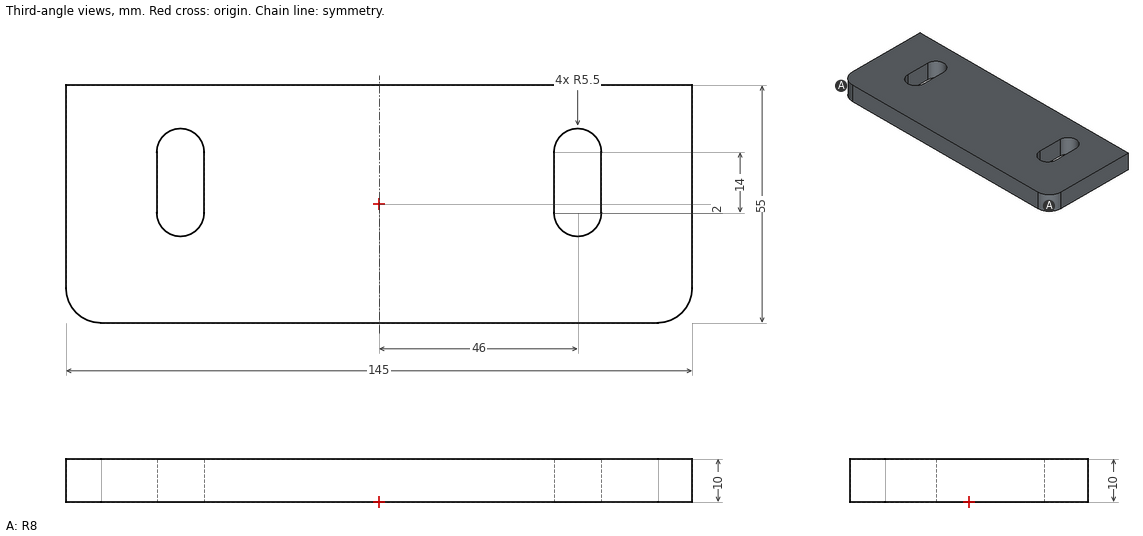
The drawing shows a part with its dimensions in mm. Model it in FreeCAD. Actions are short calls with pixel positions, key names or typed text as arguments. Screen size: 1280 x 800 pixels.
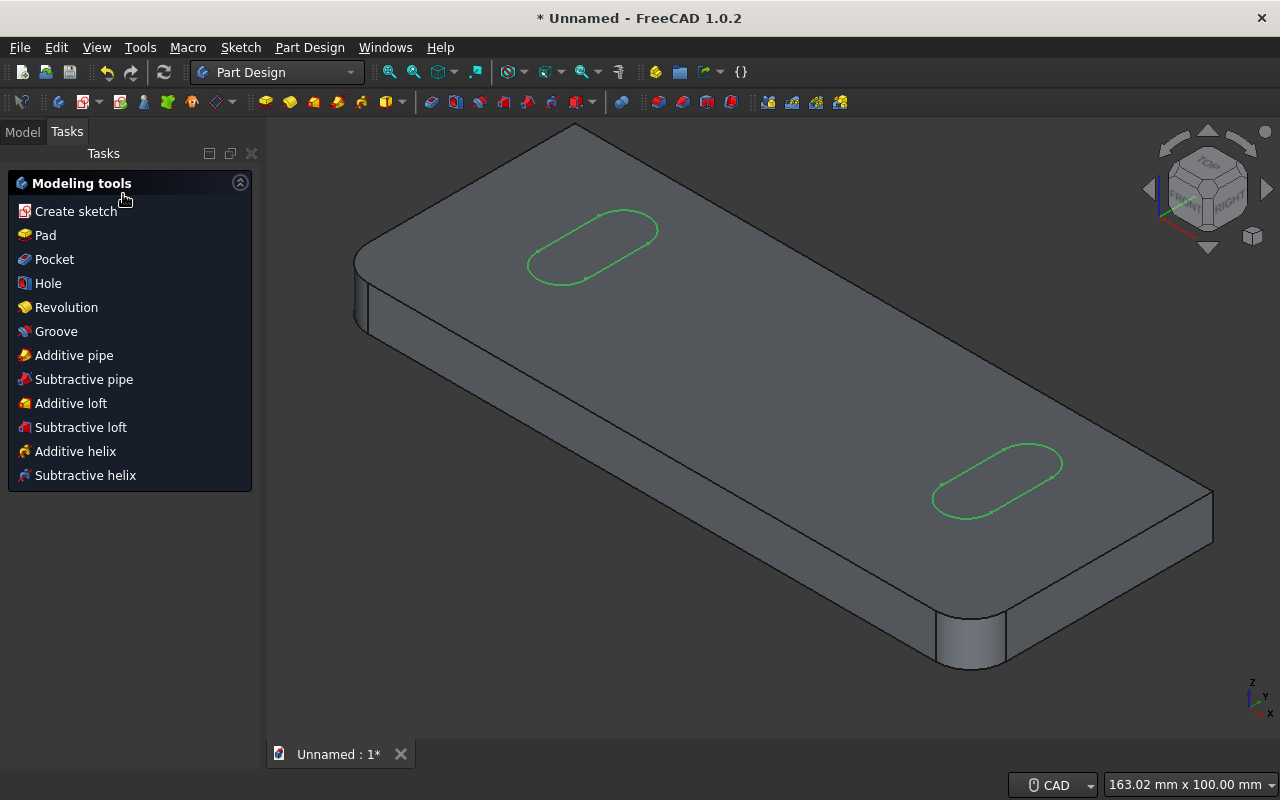
click(432, 102)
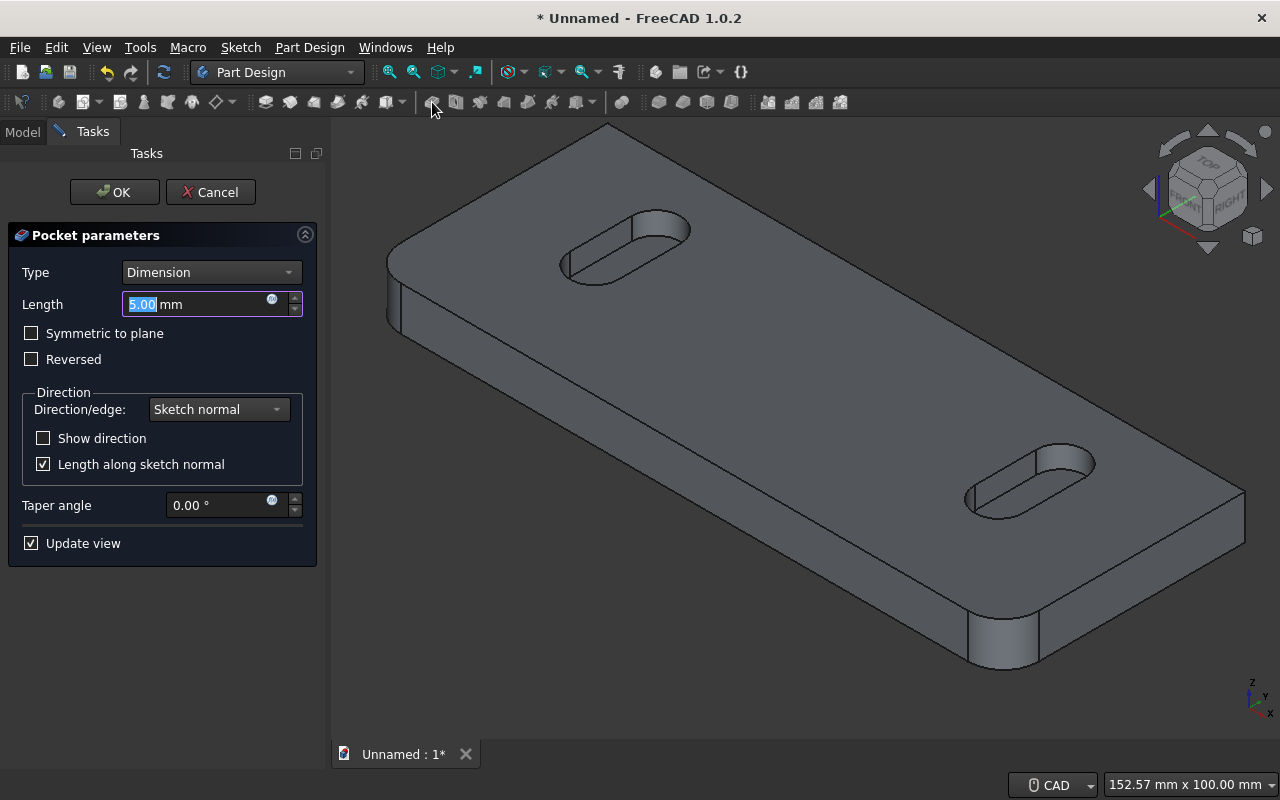
text(10)
key(Tab)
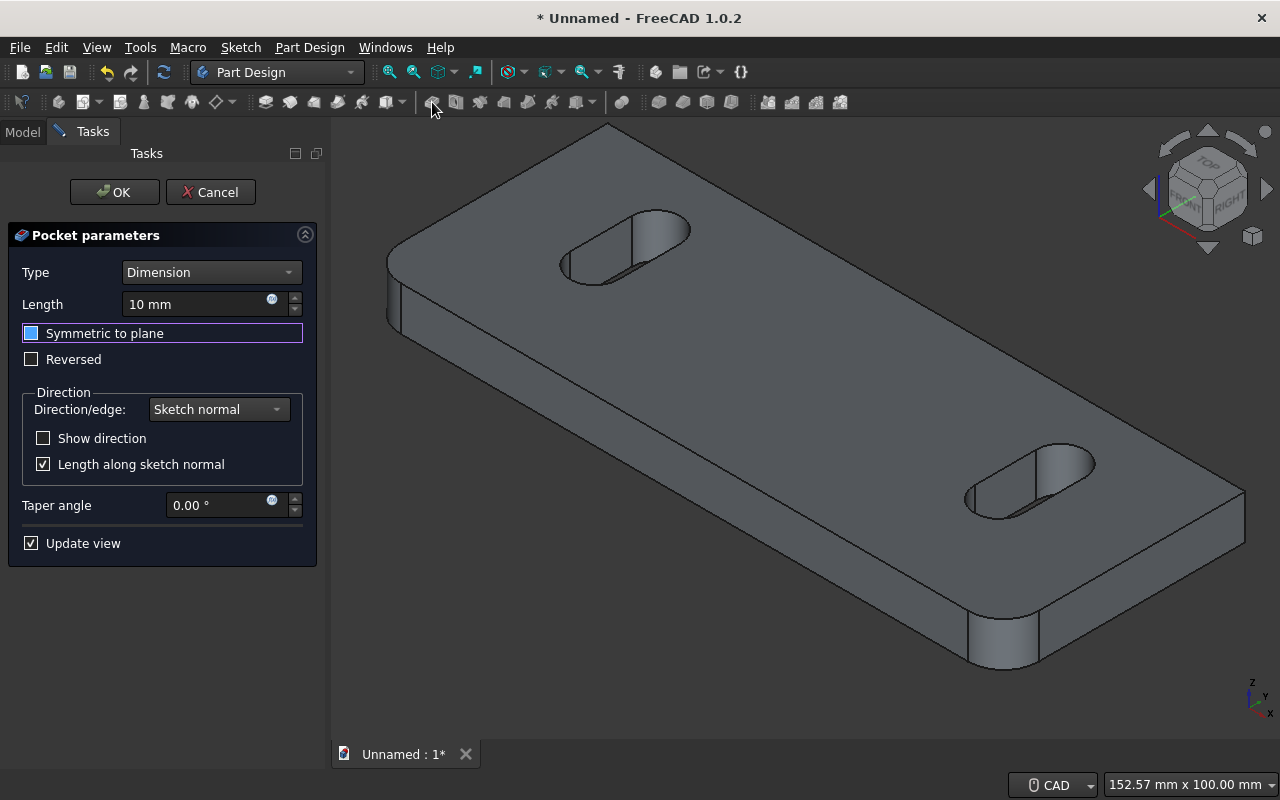
click(115, 192)